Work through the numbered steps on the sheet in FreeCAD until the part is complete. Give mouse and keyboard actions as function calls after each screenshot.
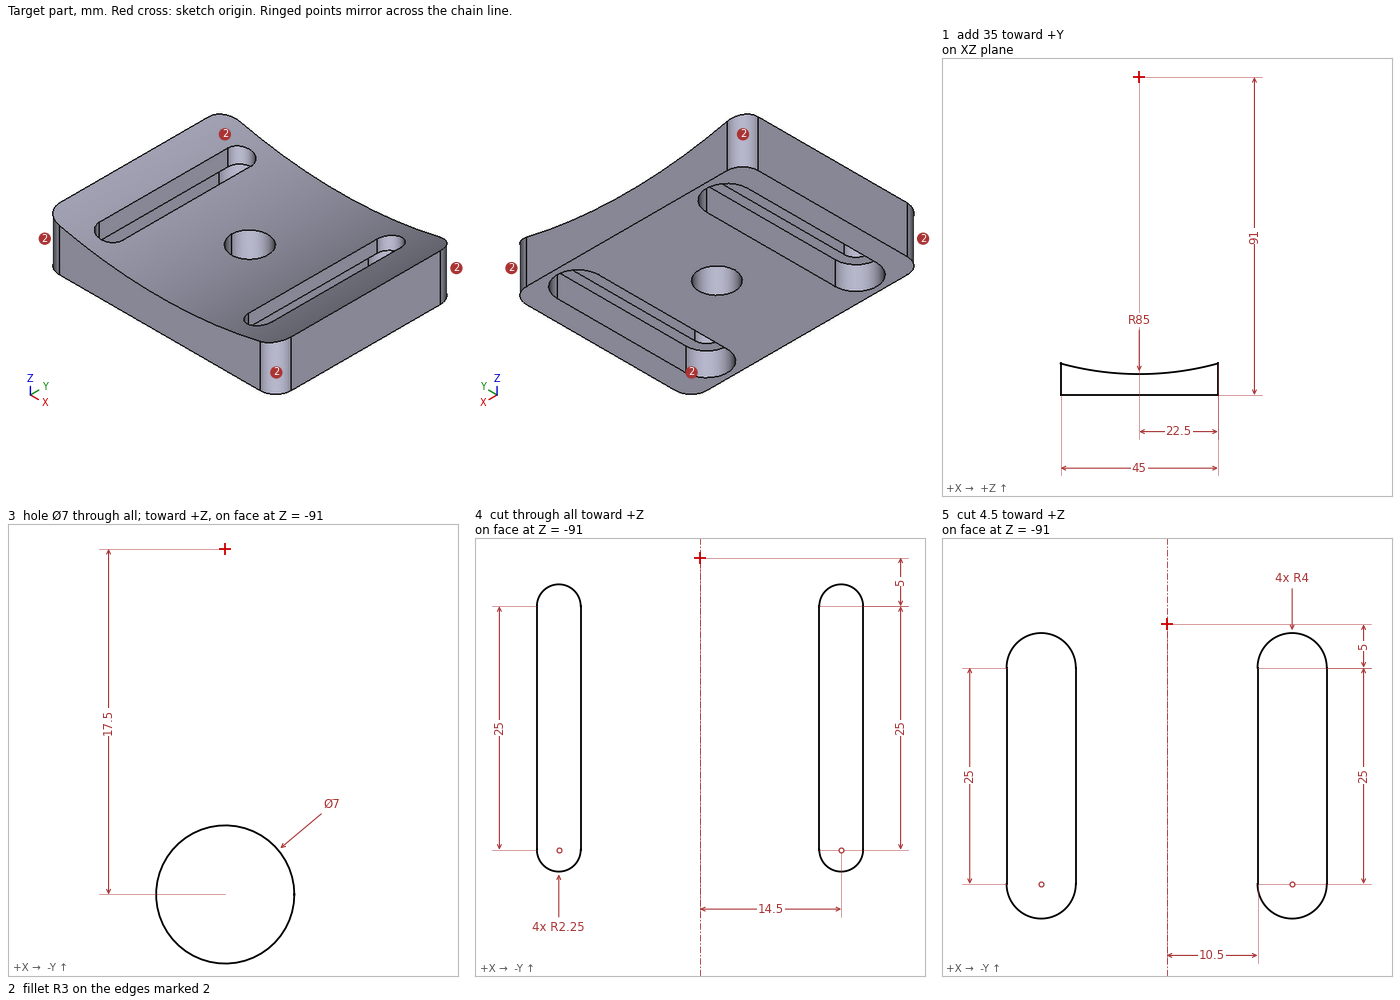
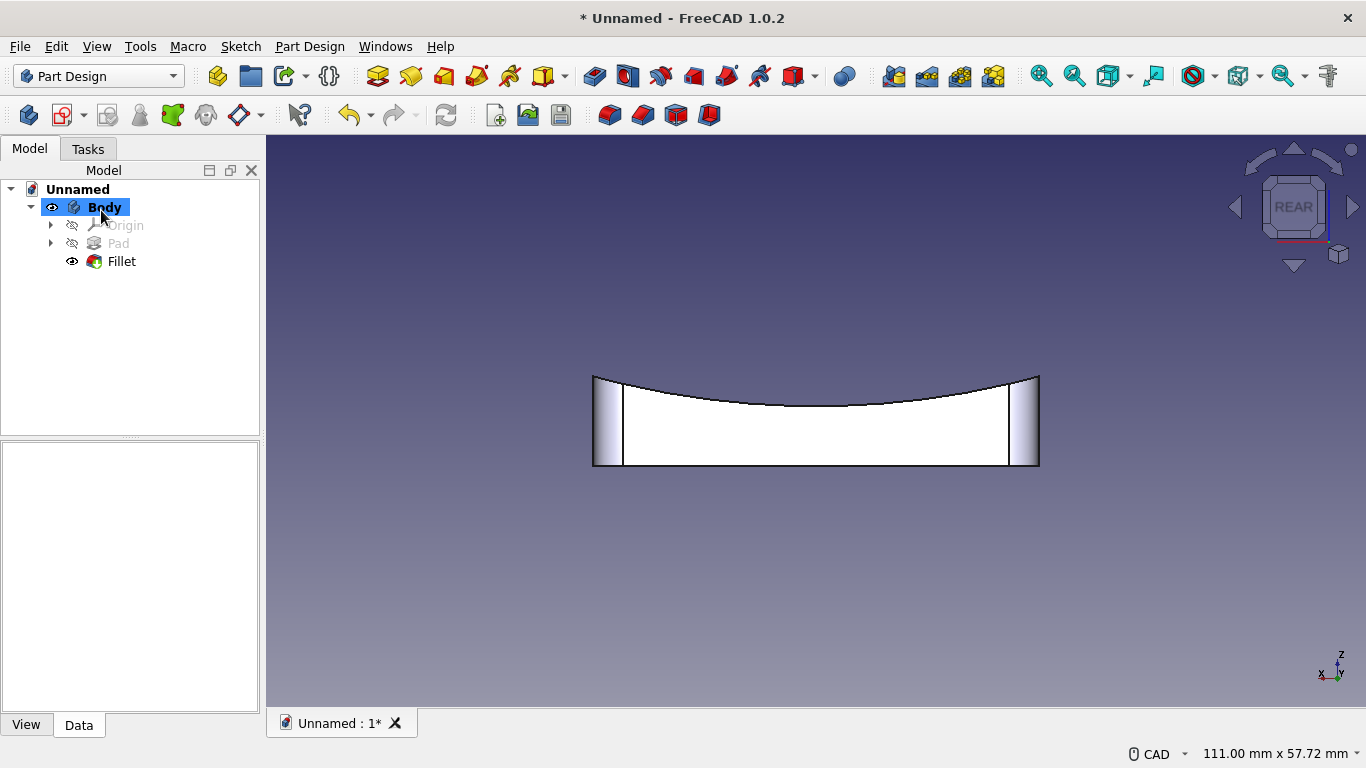
key(v)
key(f)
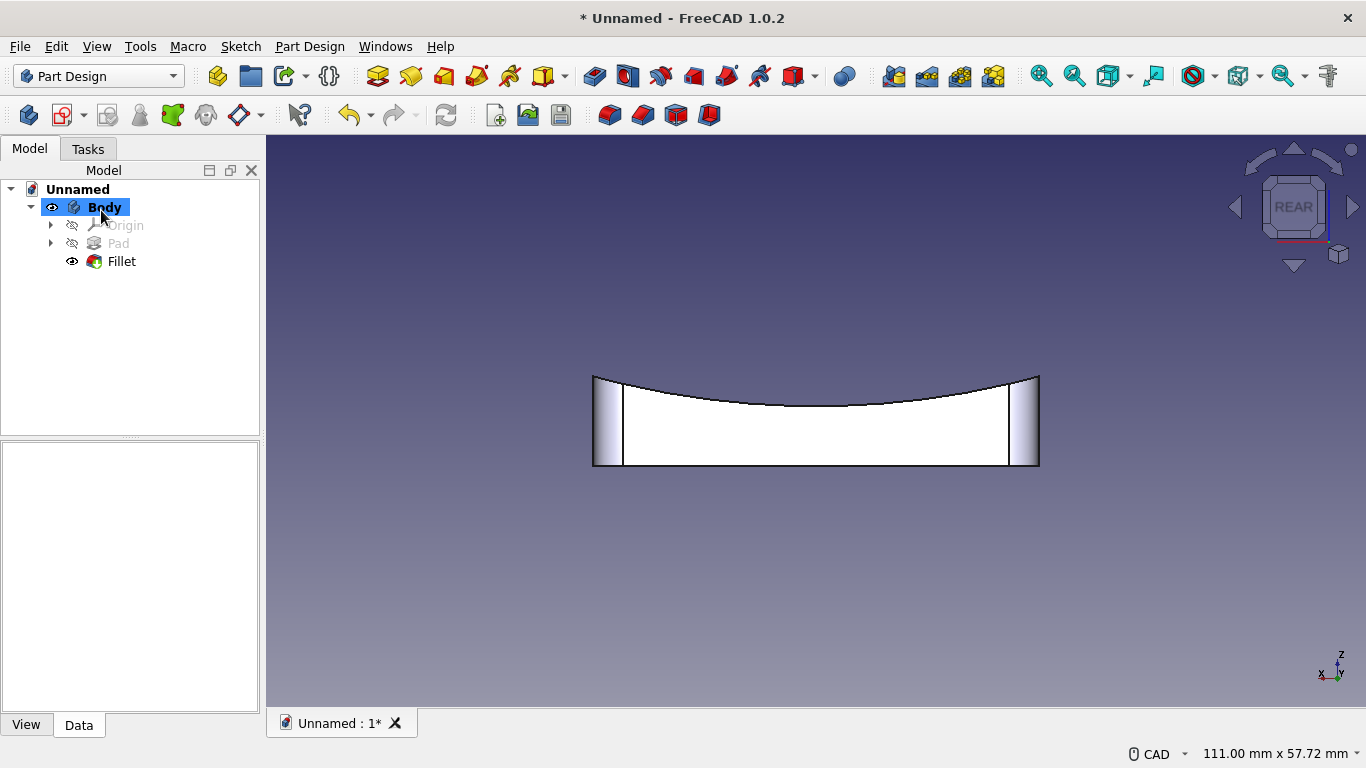
key(5)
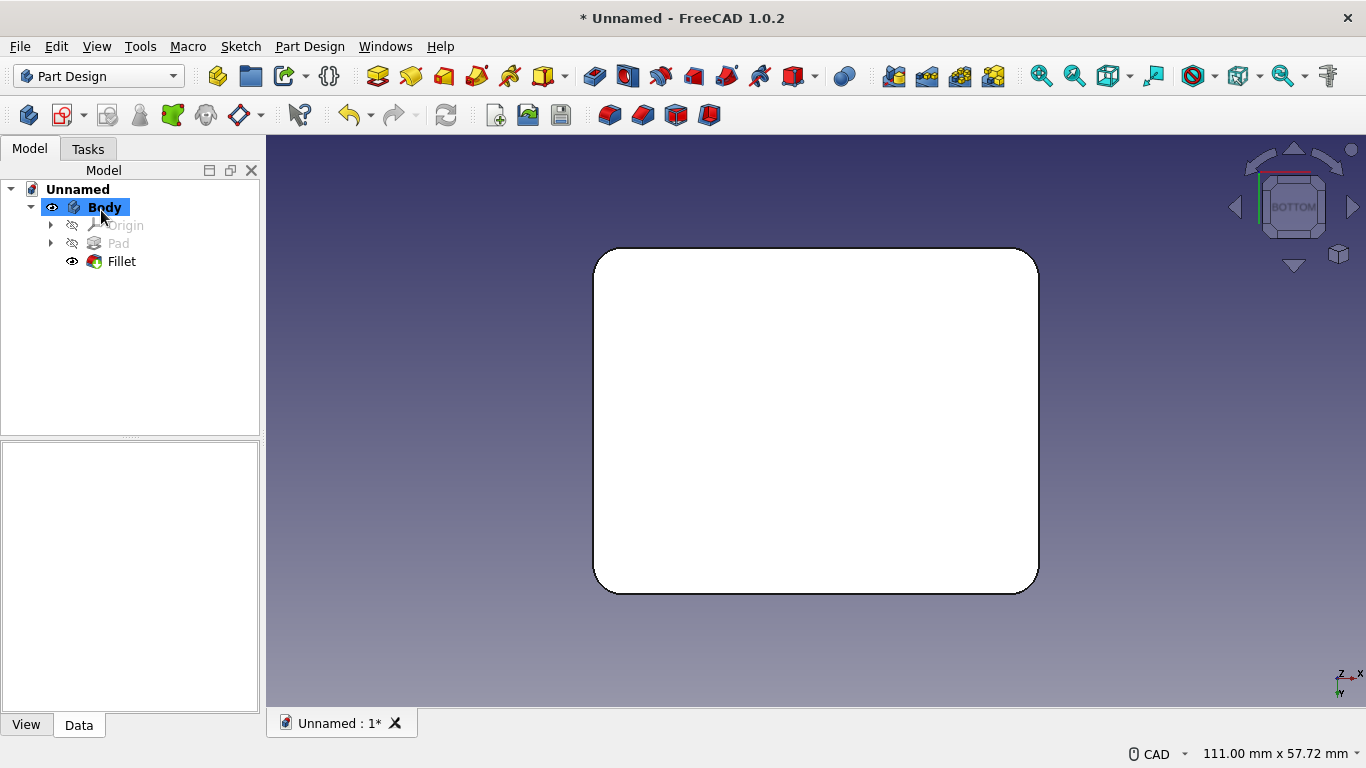
click(816, 420)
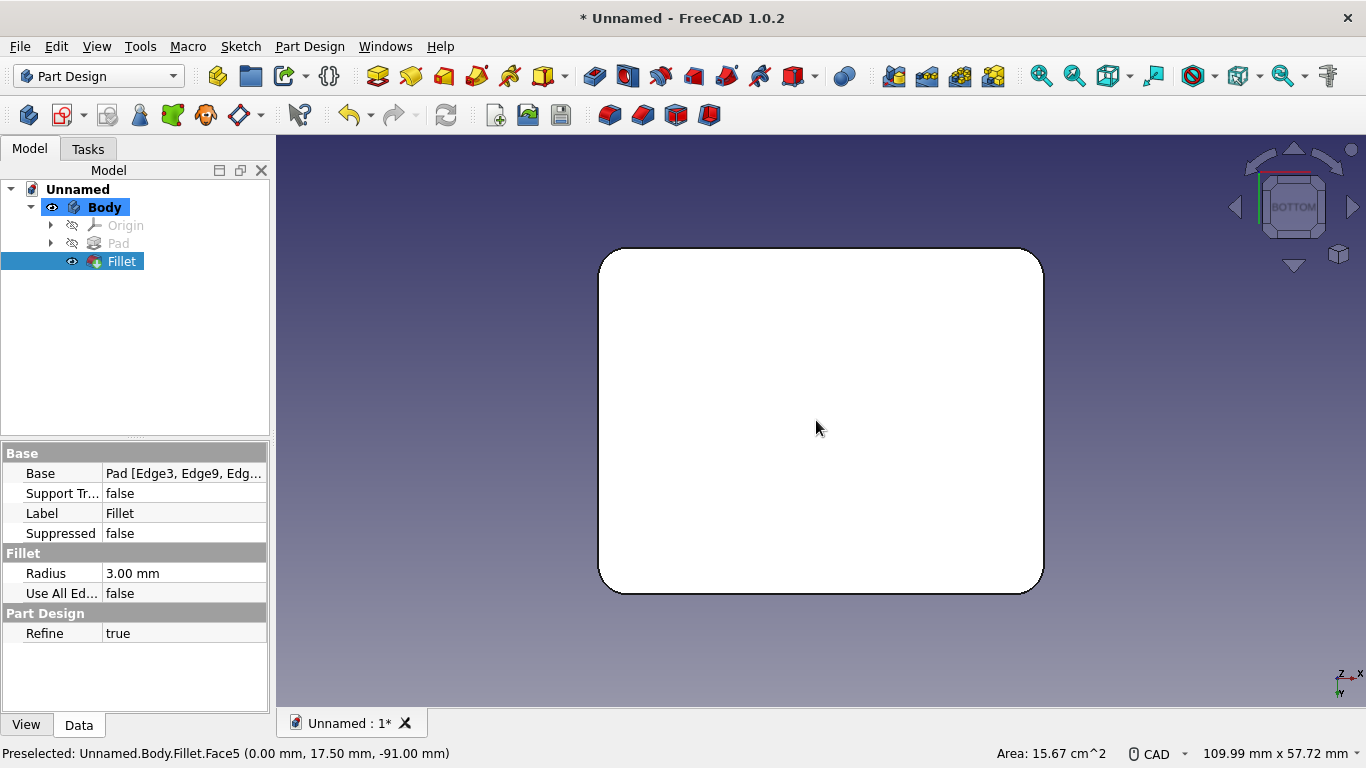
click(62, 116)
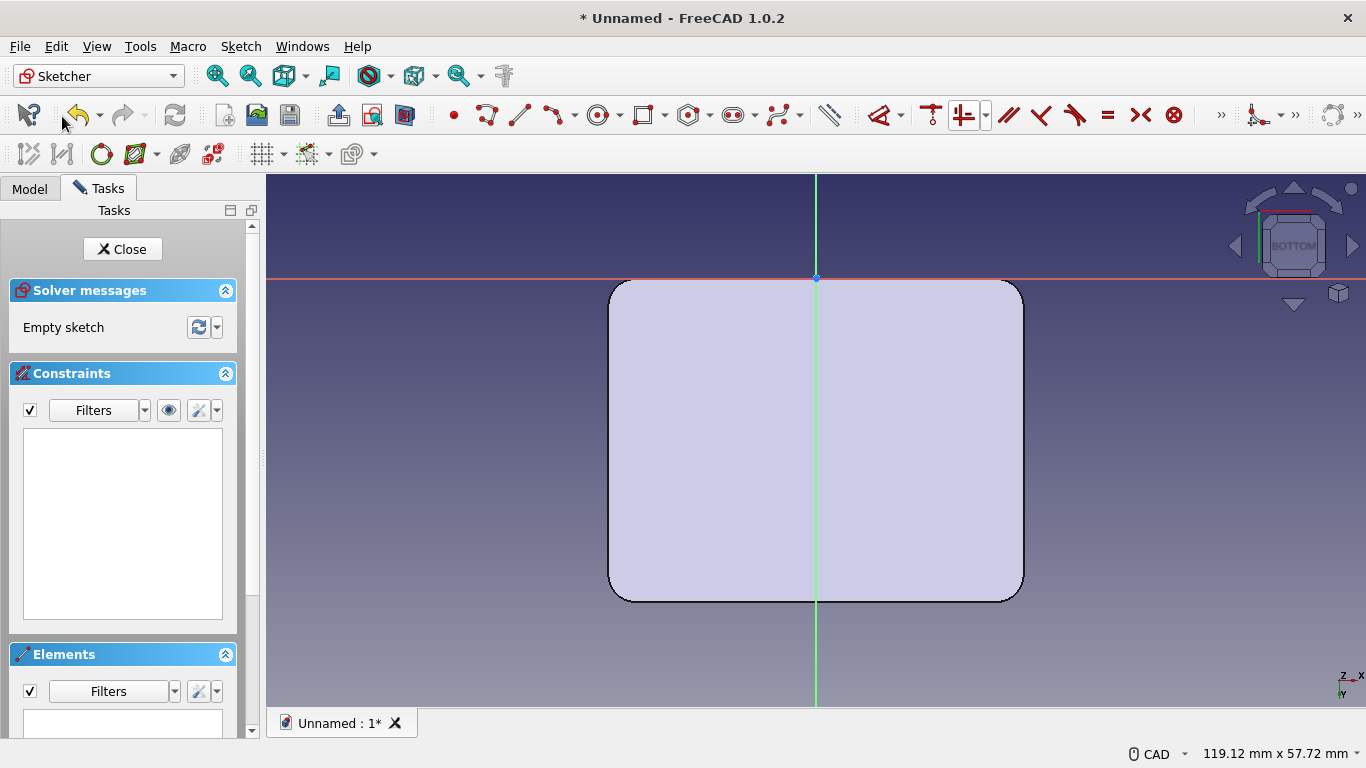
scroll(833, 440, up, 8)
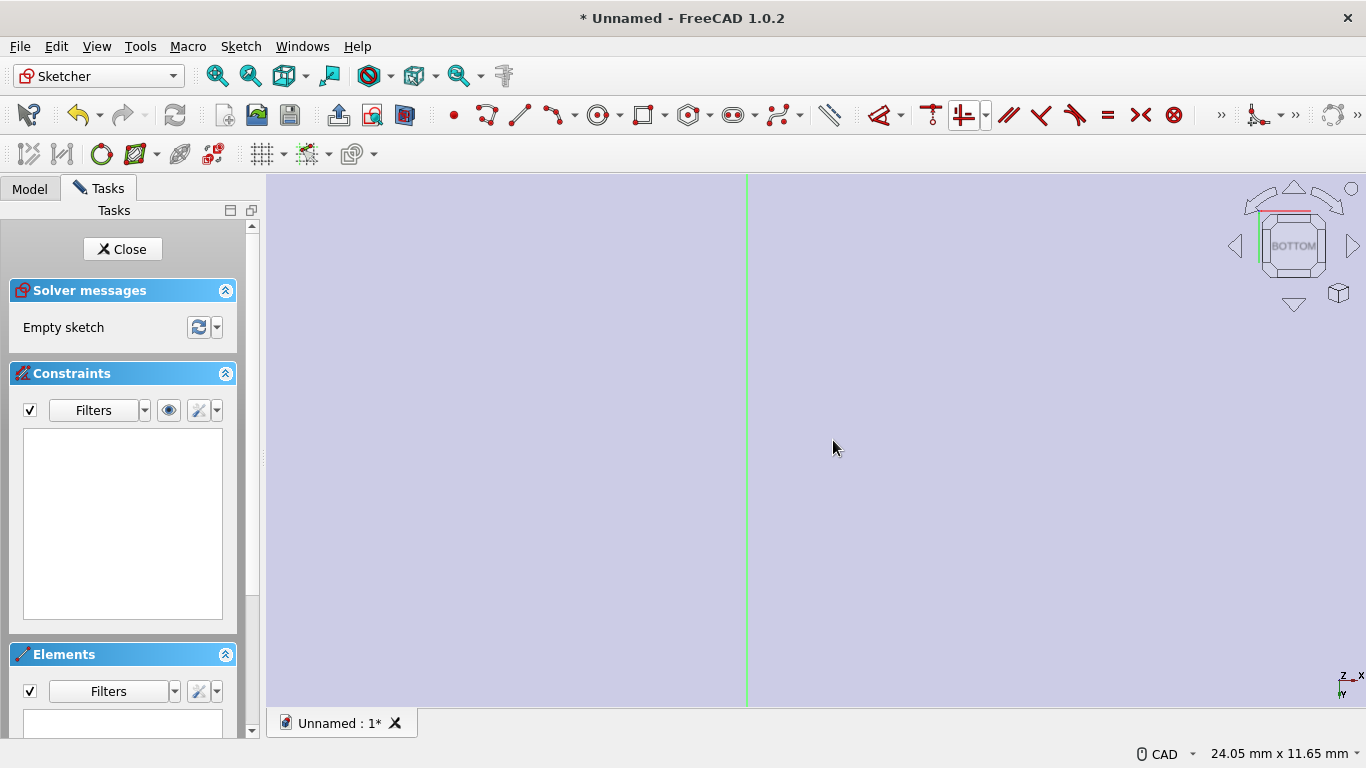
key(g)
key(c)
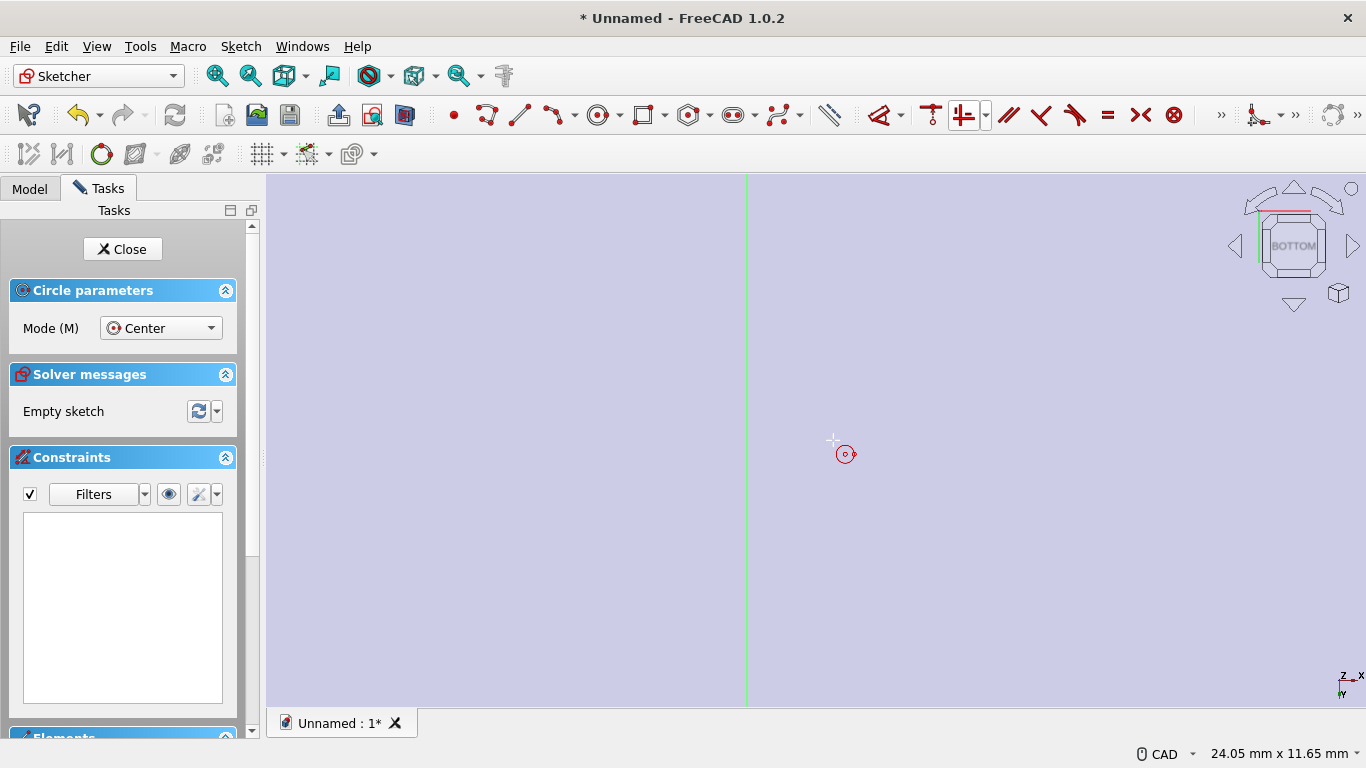
click(747, 440)
click(860, 327)
key(Escape)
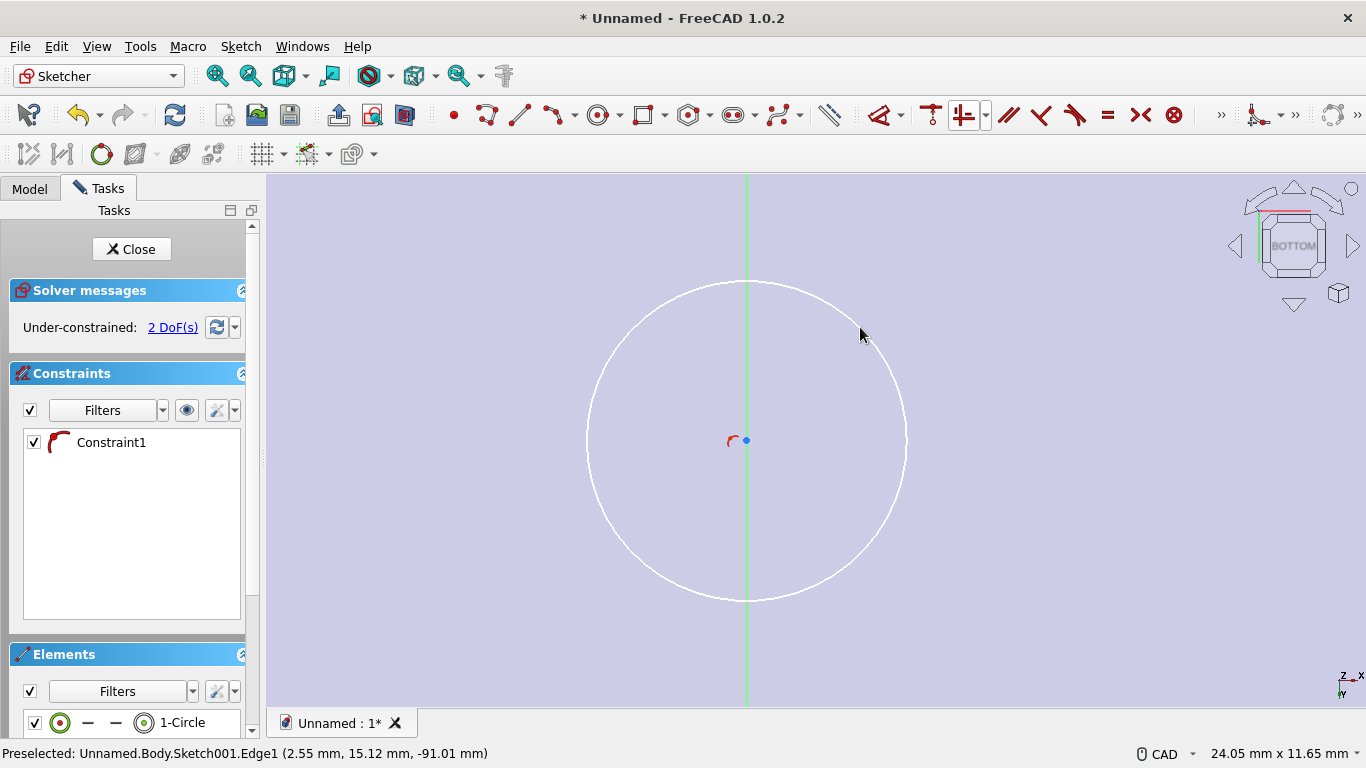
click(878, 116)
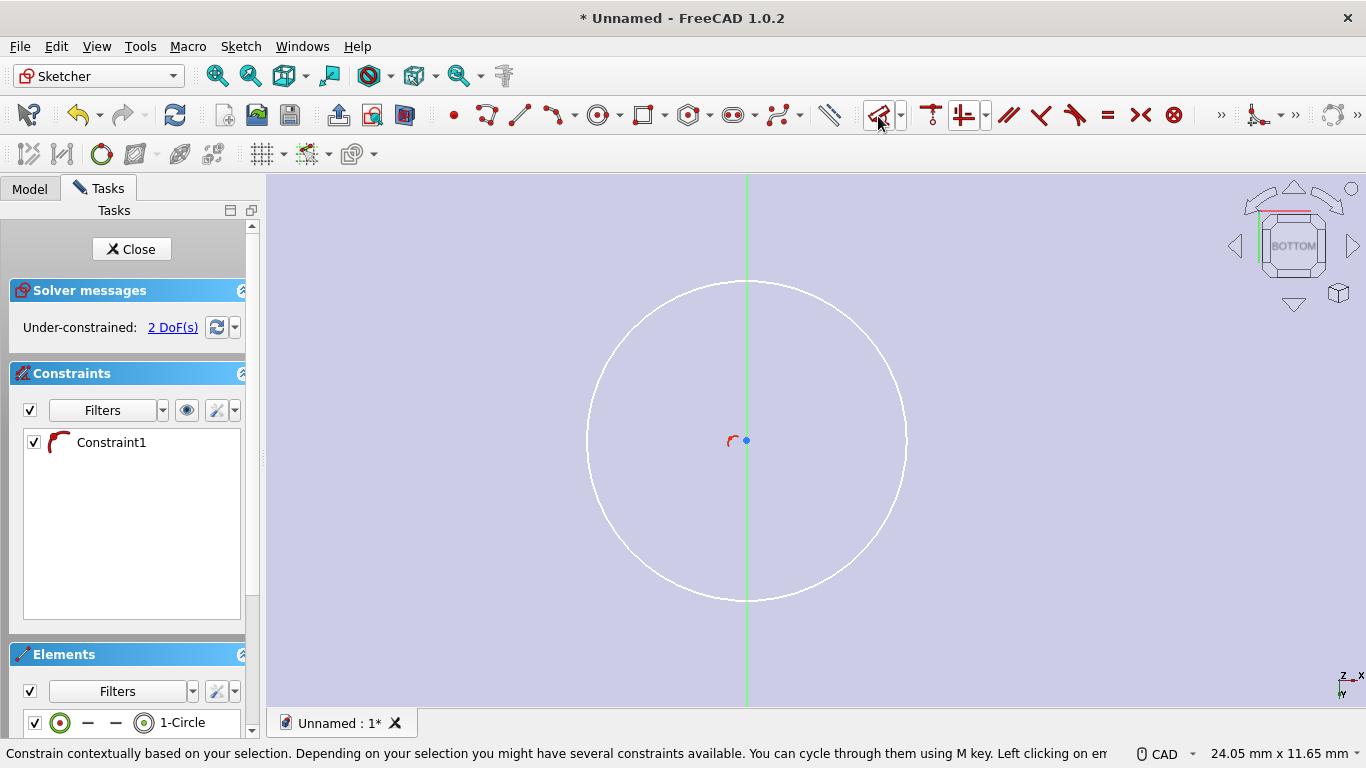
click(860, 328)
click(883, 305)